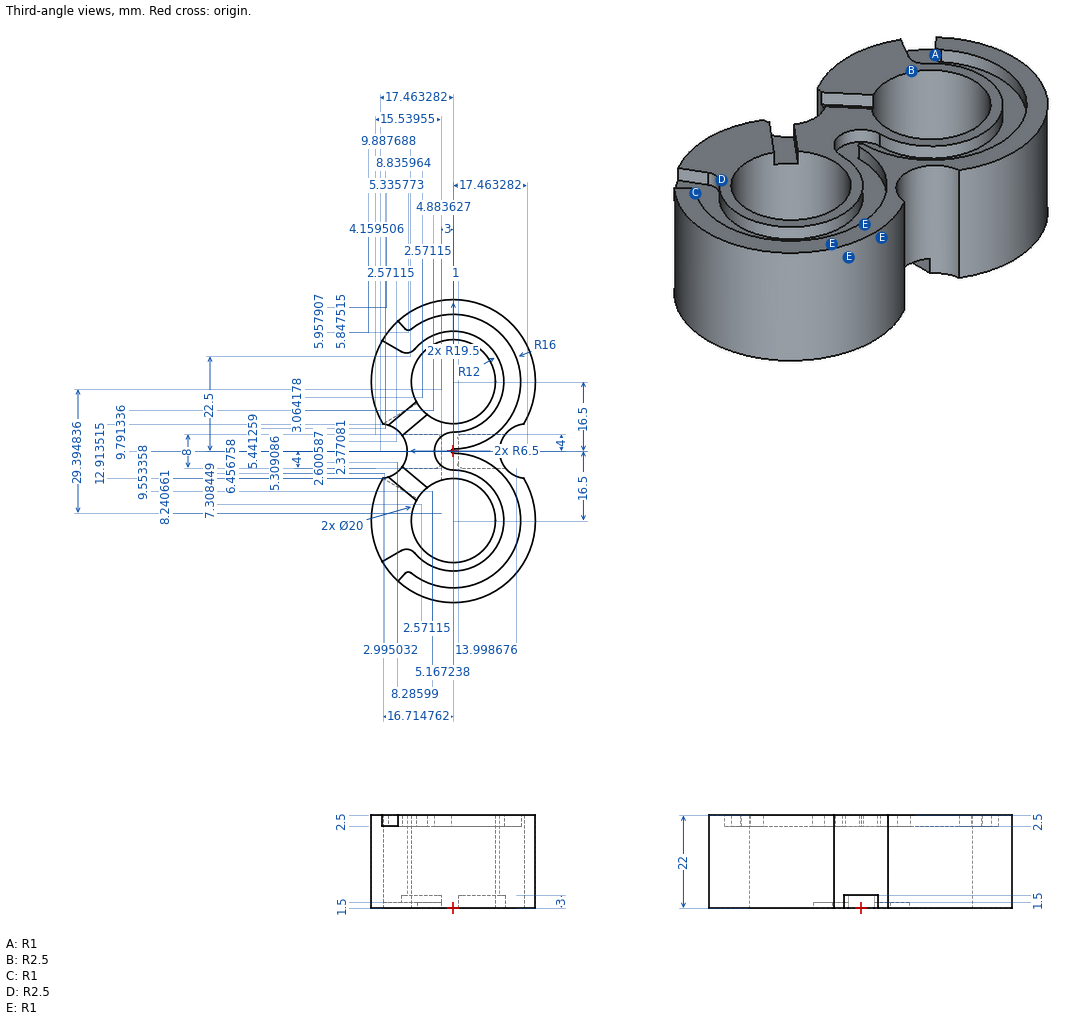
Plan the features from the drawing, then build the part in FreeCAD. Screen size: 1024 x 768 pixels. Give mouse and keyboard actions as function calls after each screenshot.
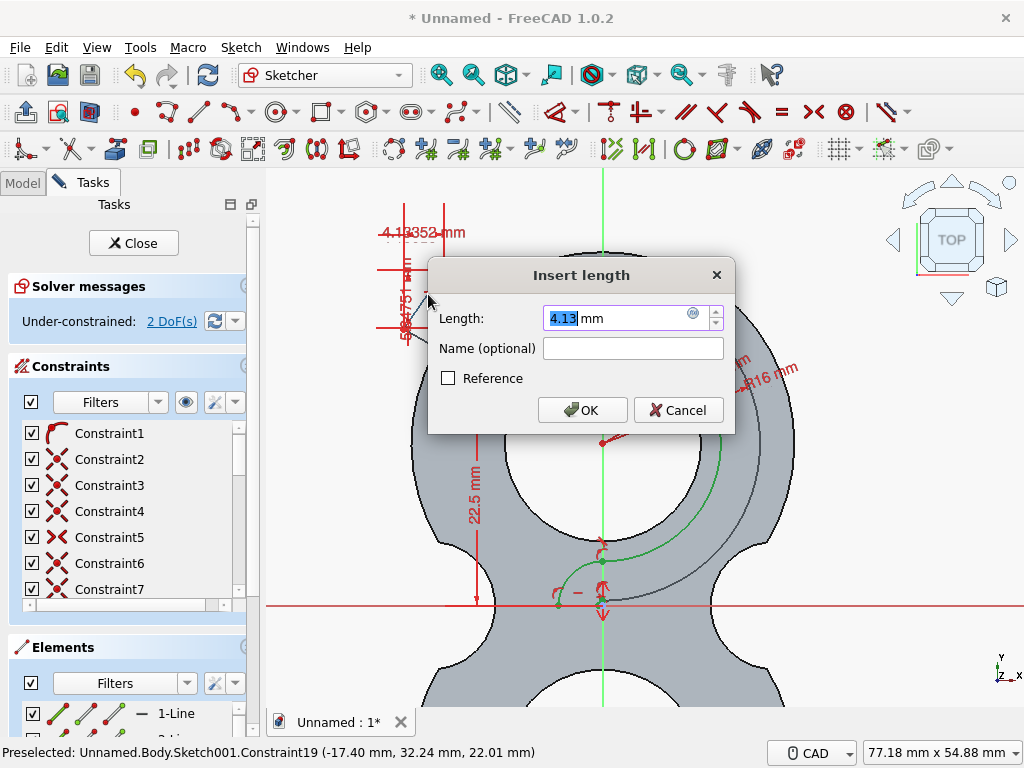
text(4.159506)
key(Return)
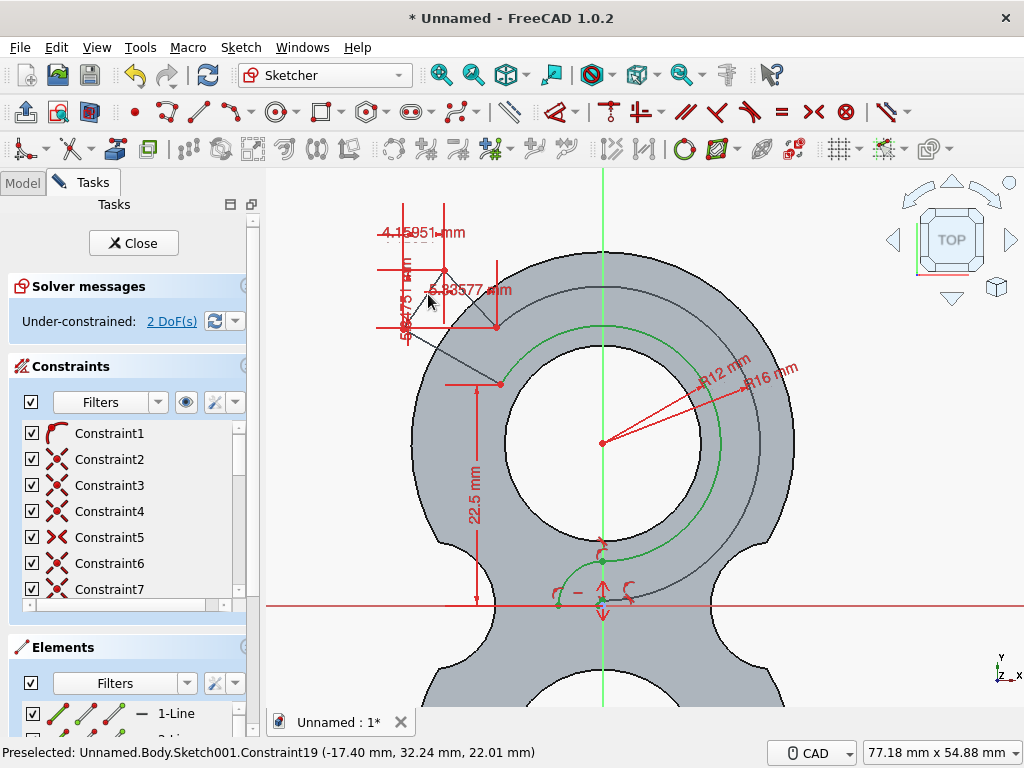
click(428, 294)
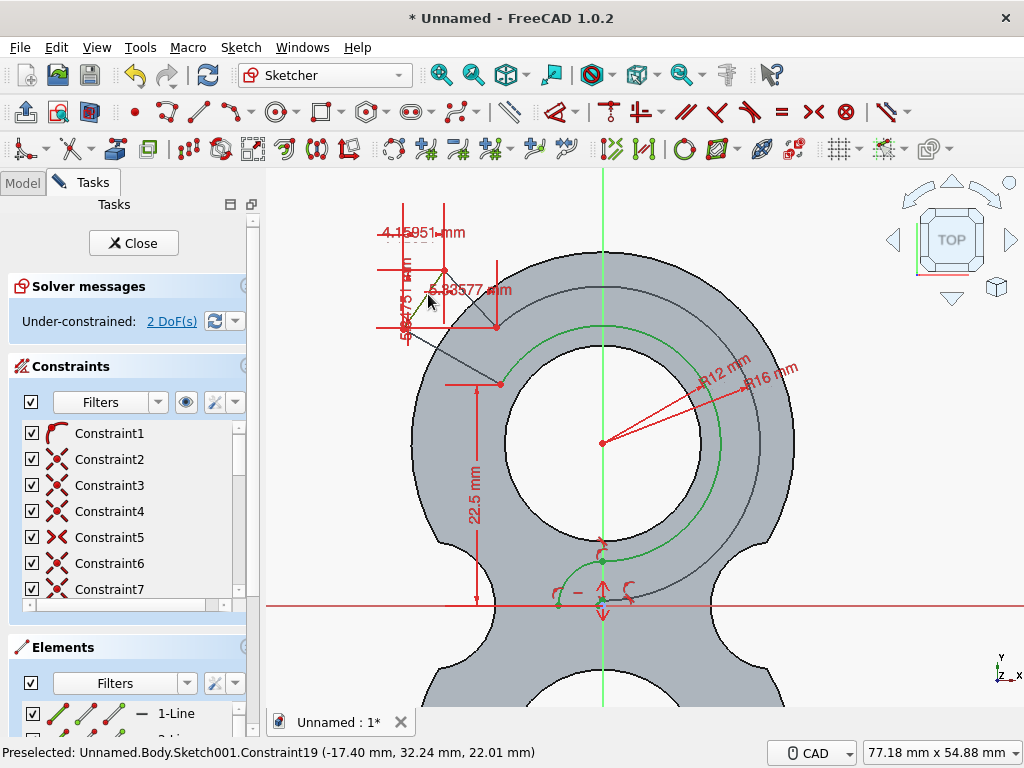
key(i)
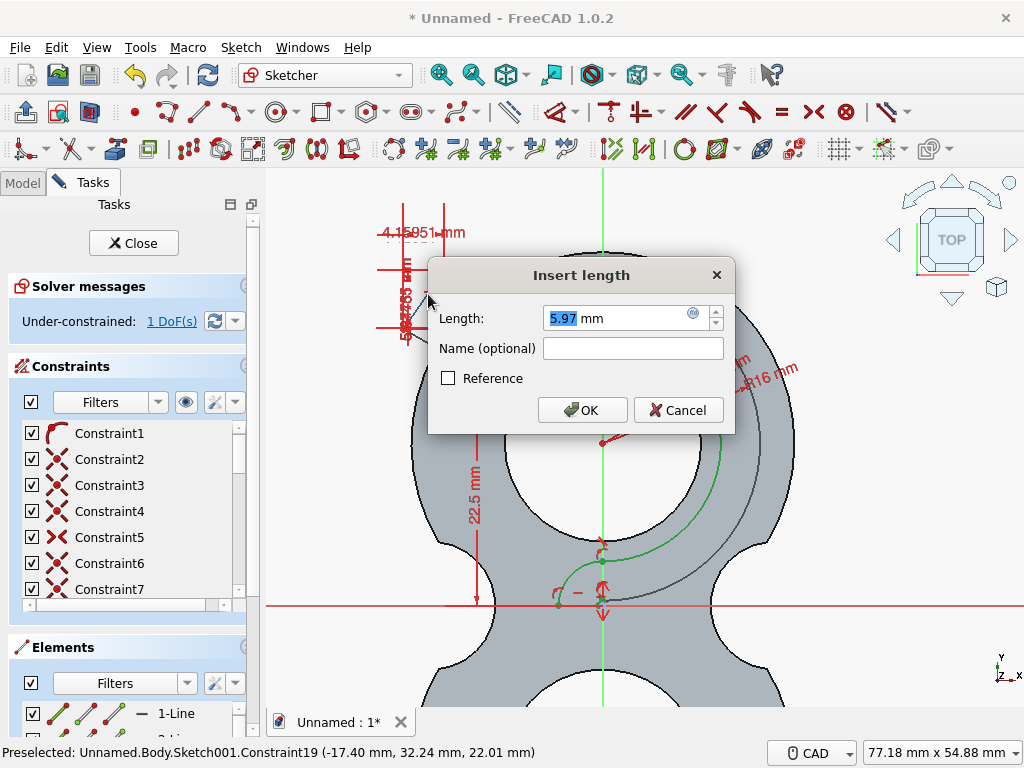
text(5.957907)
key(Return)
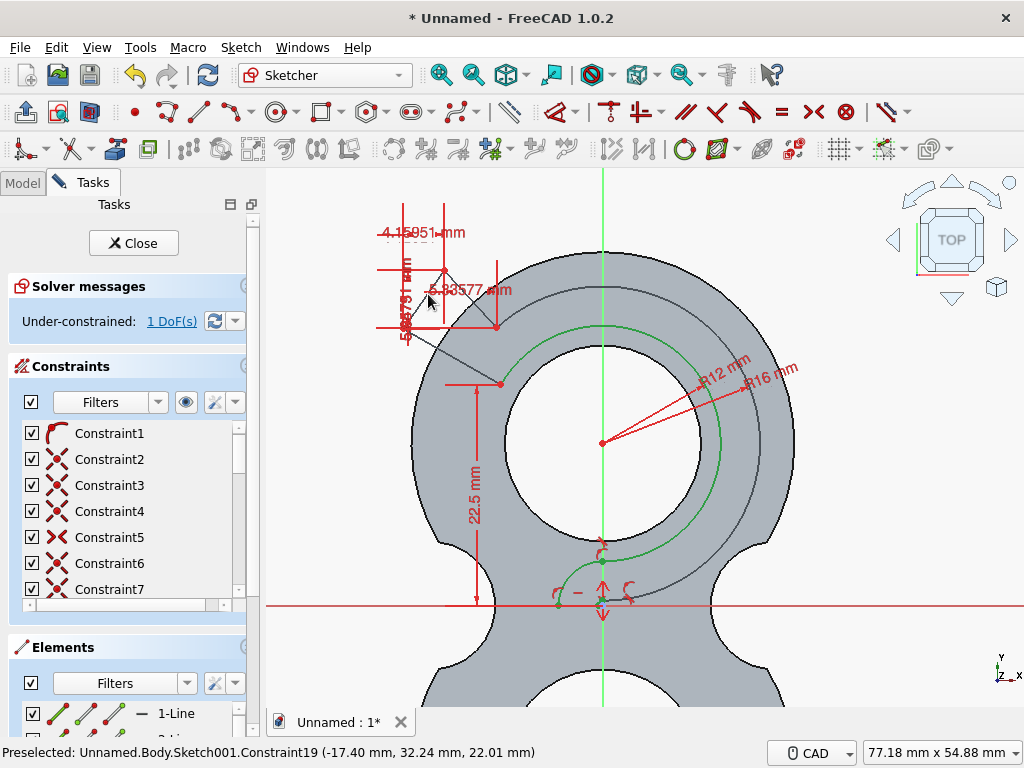
click(433, 346)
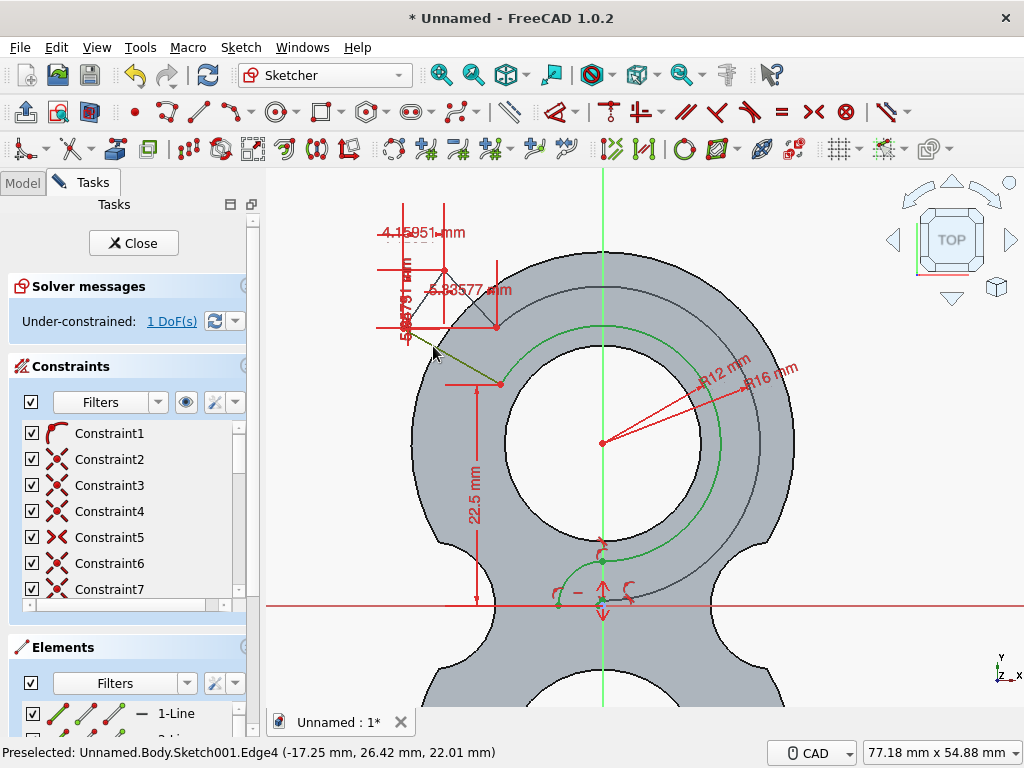
key(l)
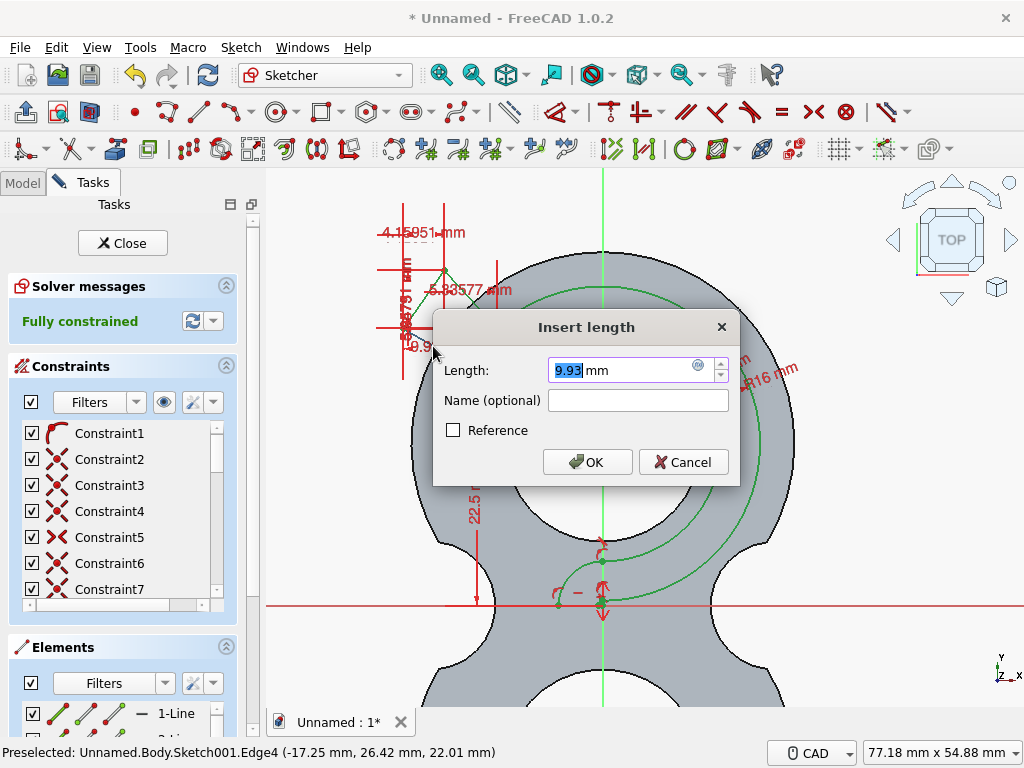
text(9.887688)
key(Return)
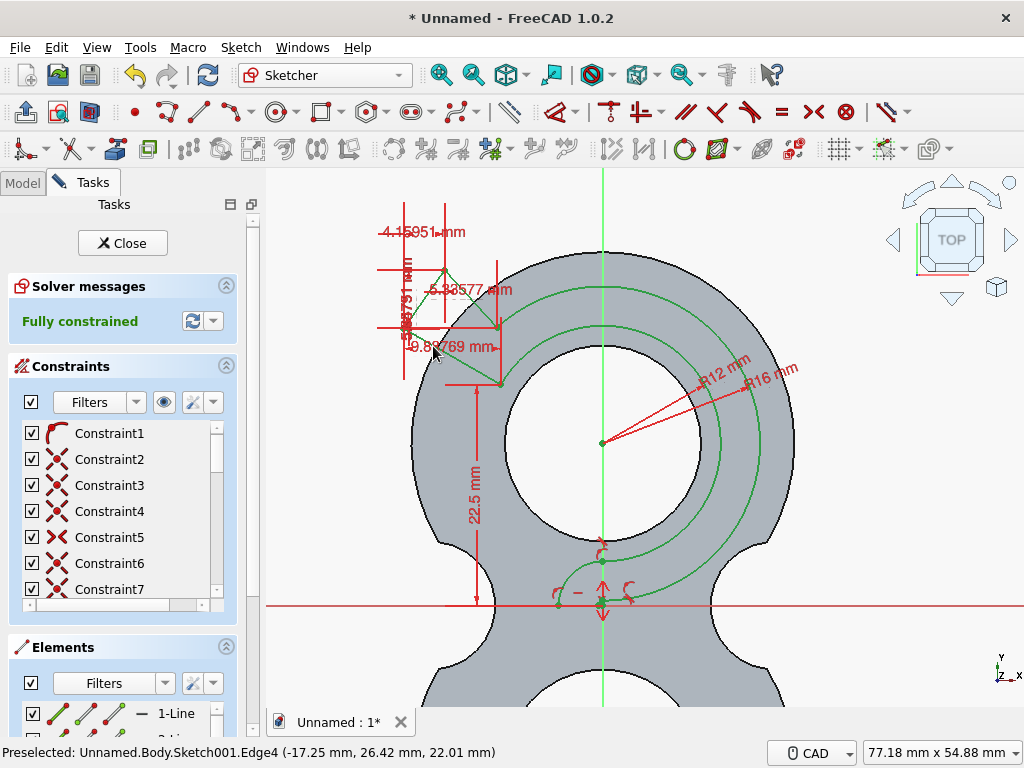
click(123, 243)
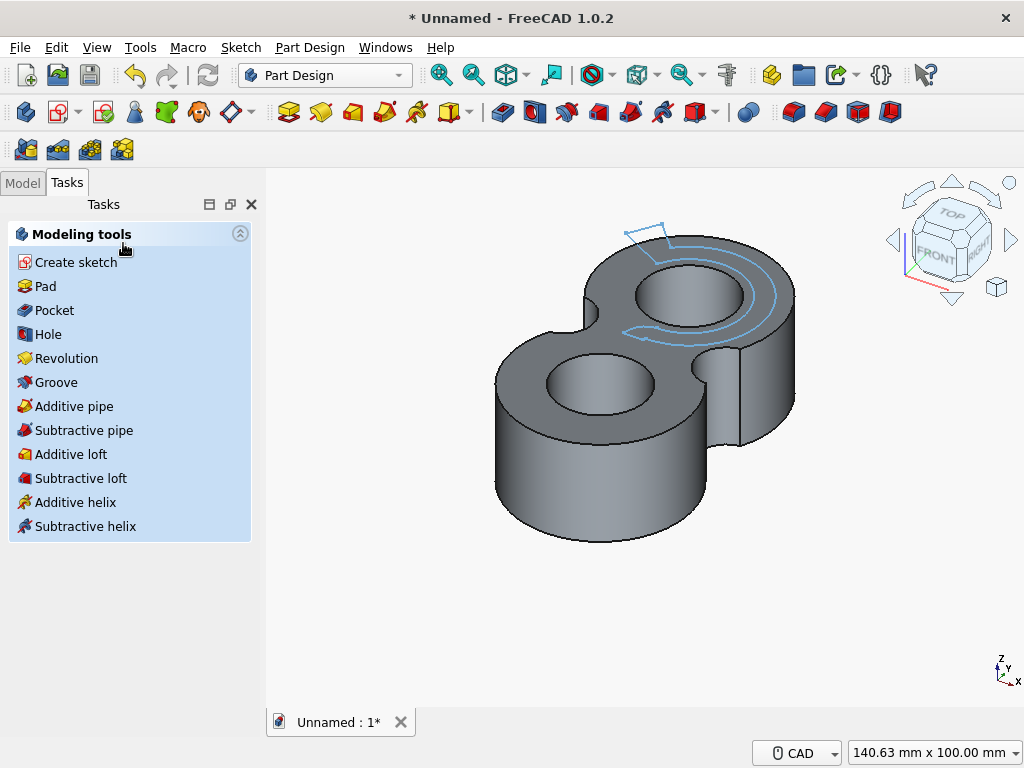
click(504, 112)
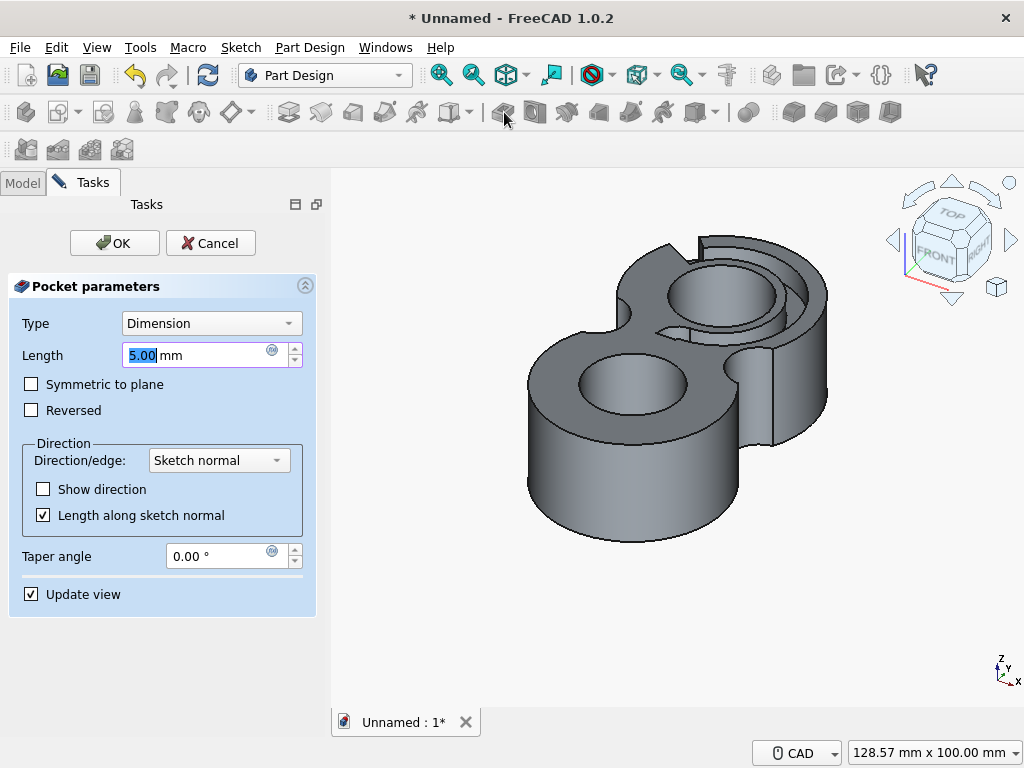
text(2.5)
key(Tab)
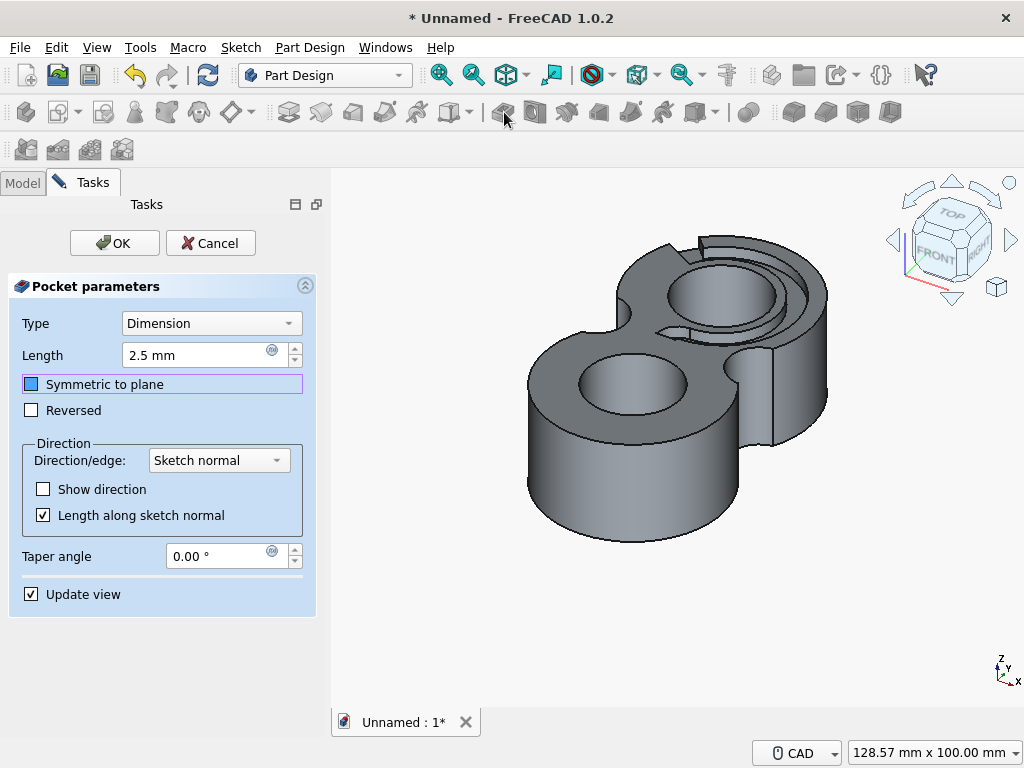
click(115, 243)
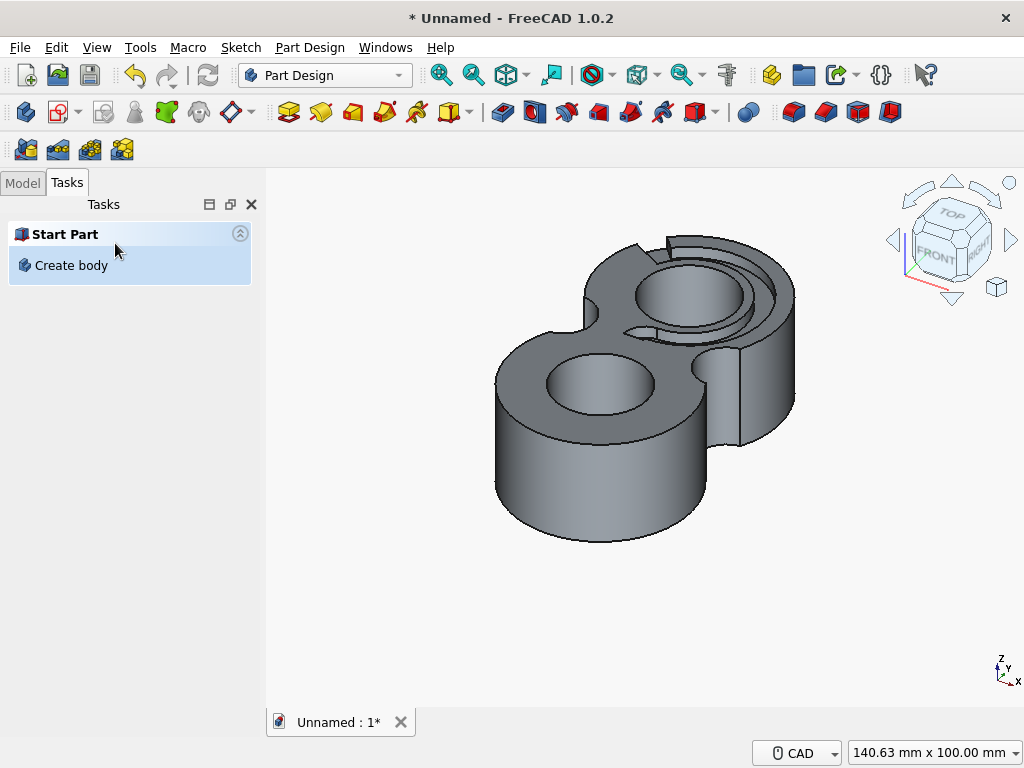
click(671, 253)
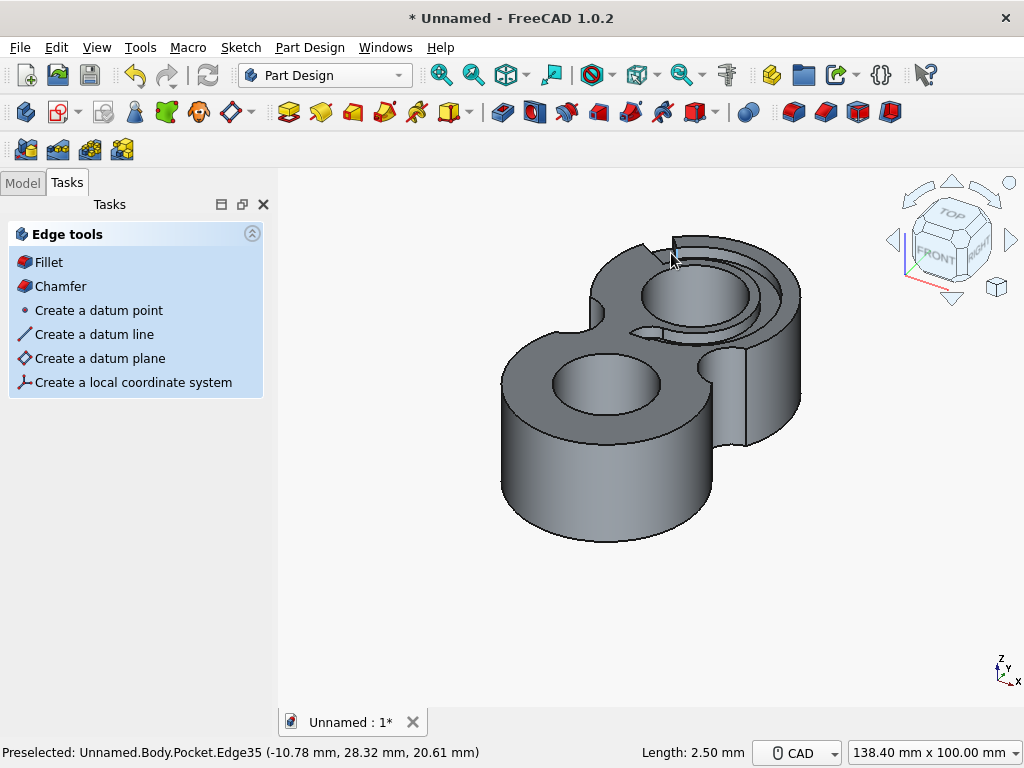
click(794, 112)